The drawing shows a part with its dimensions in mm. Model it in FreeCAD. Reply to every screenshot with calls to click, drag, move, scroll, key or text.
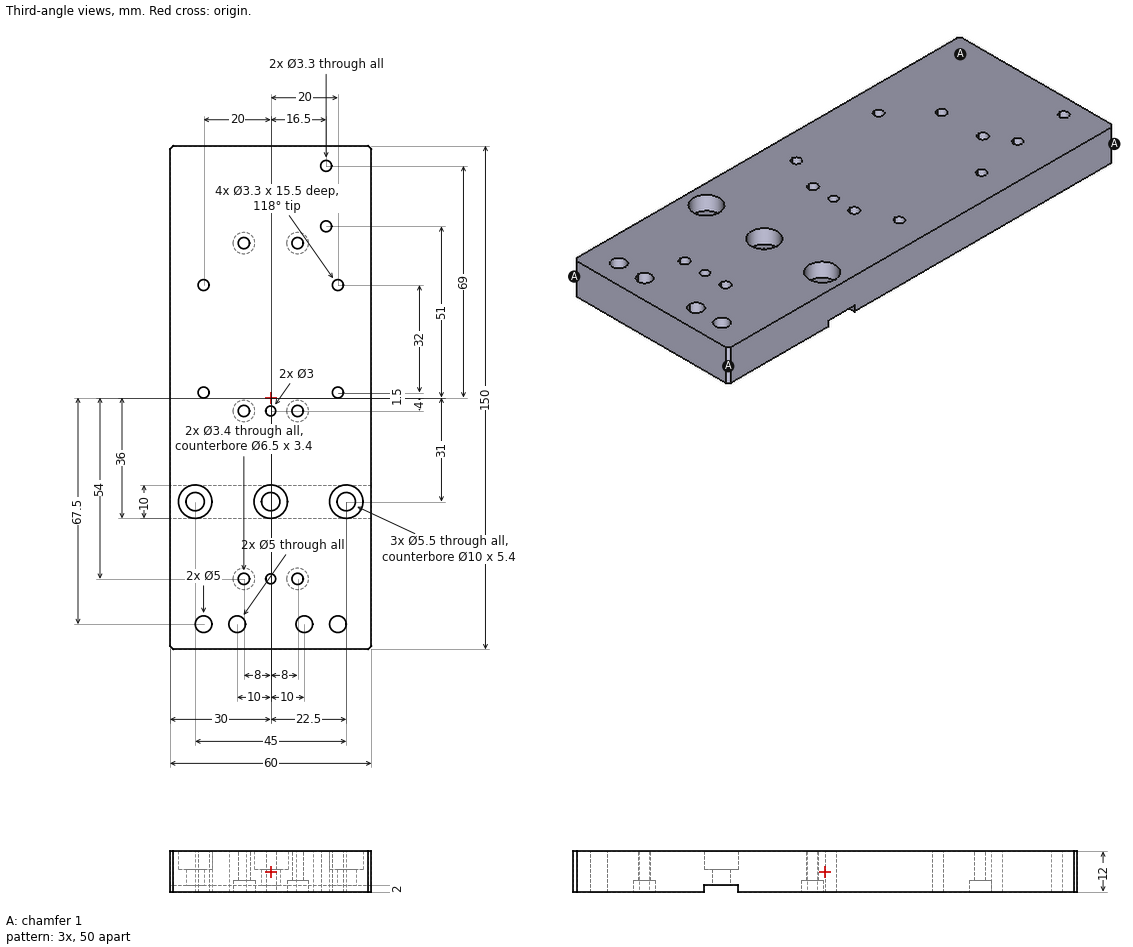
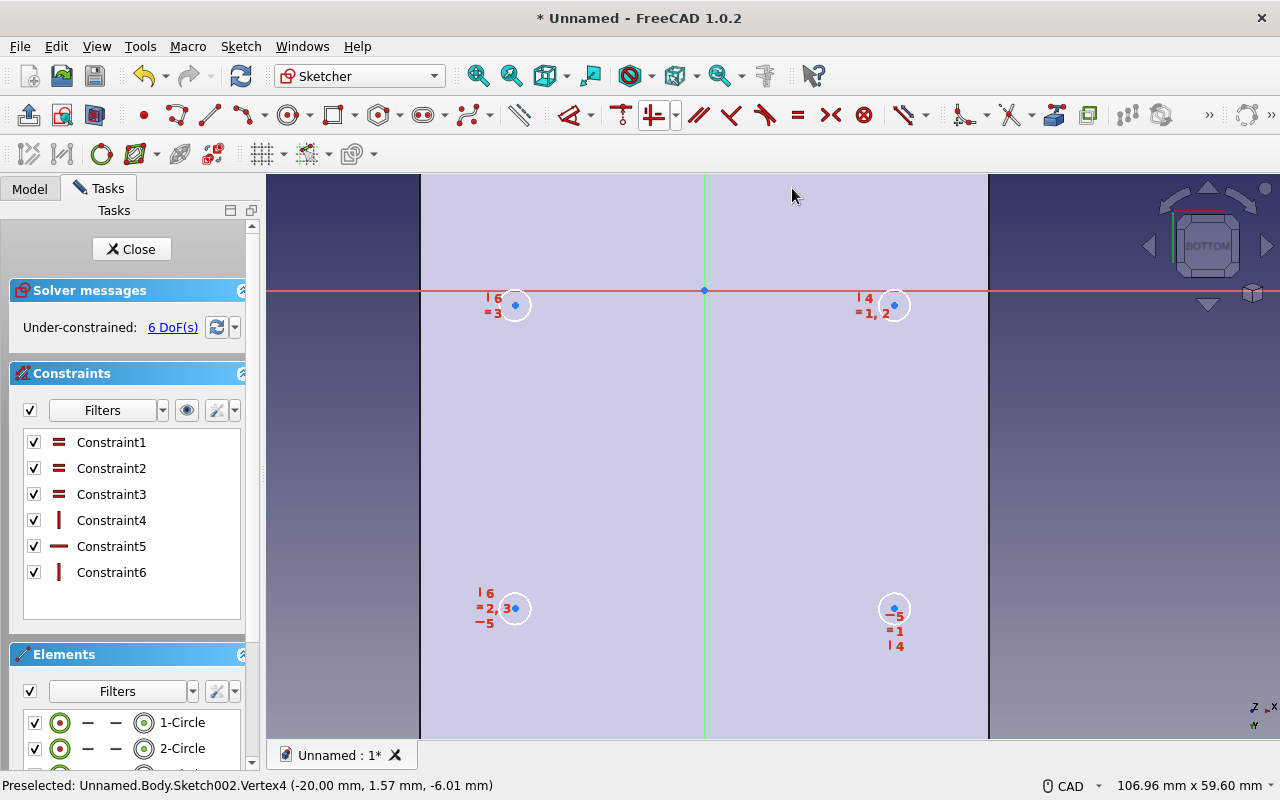
click(895, 305)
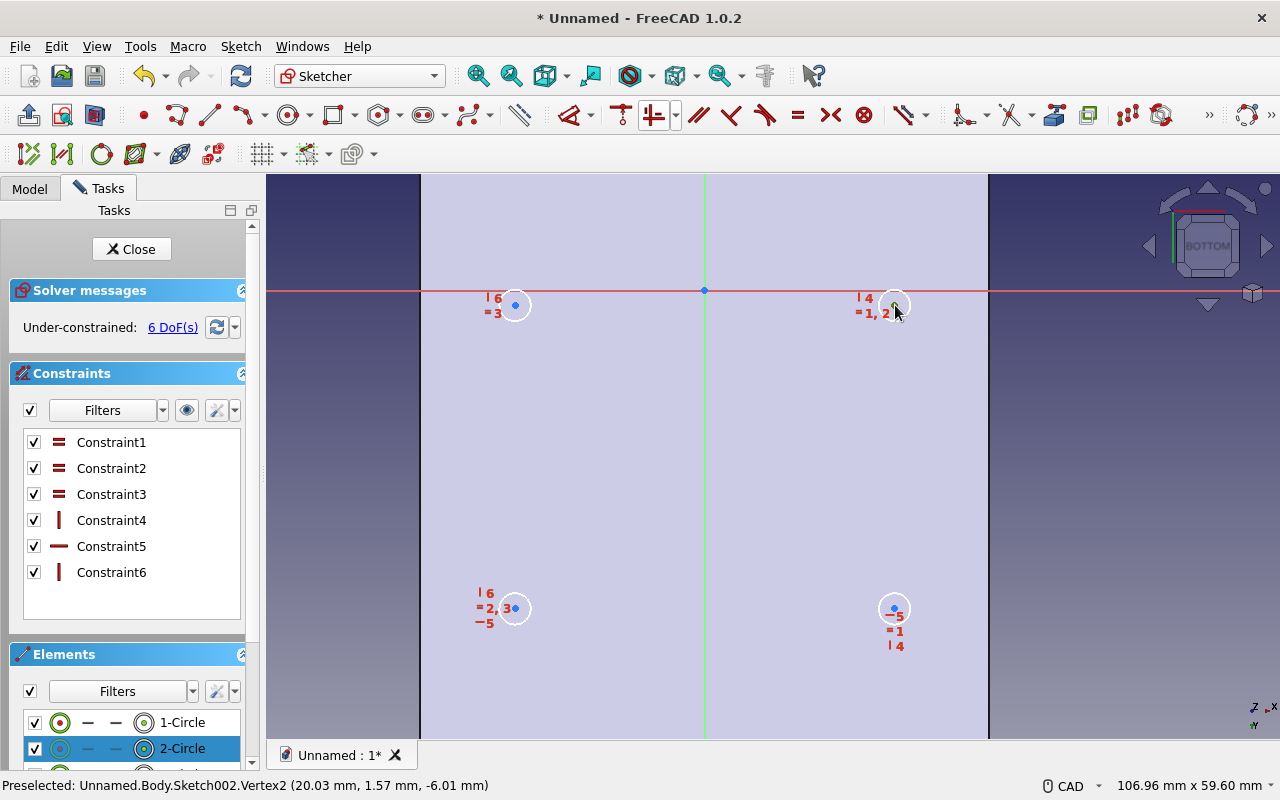
click(515, 305)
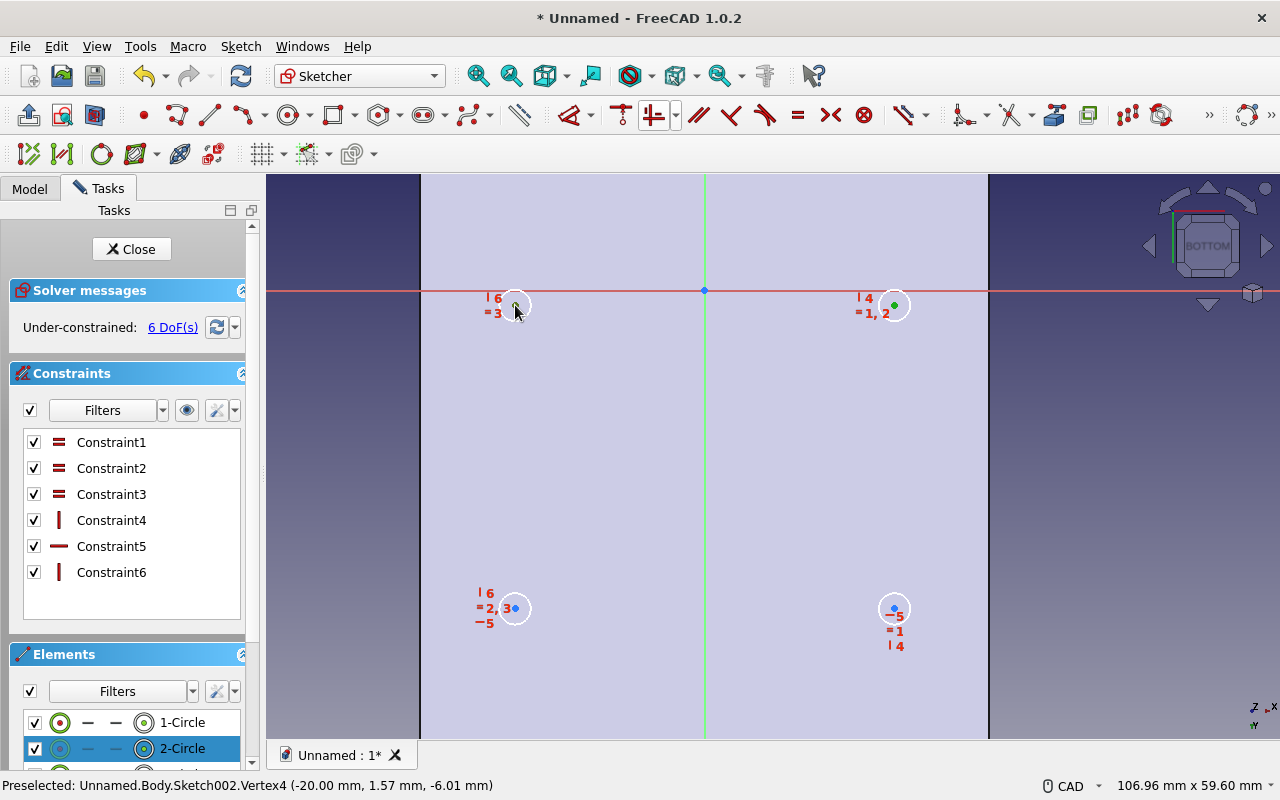
click(676, 116)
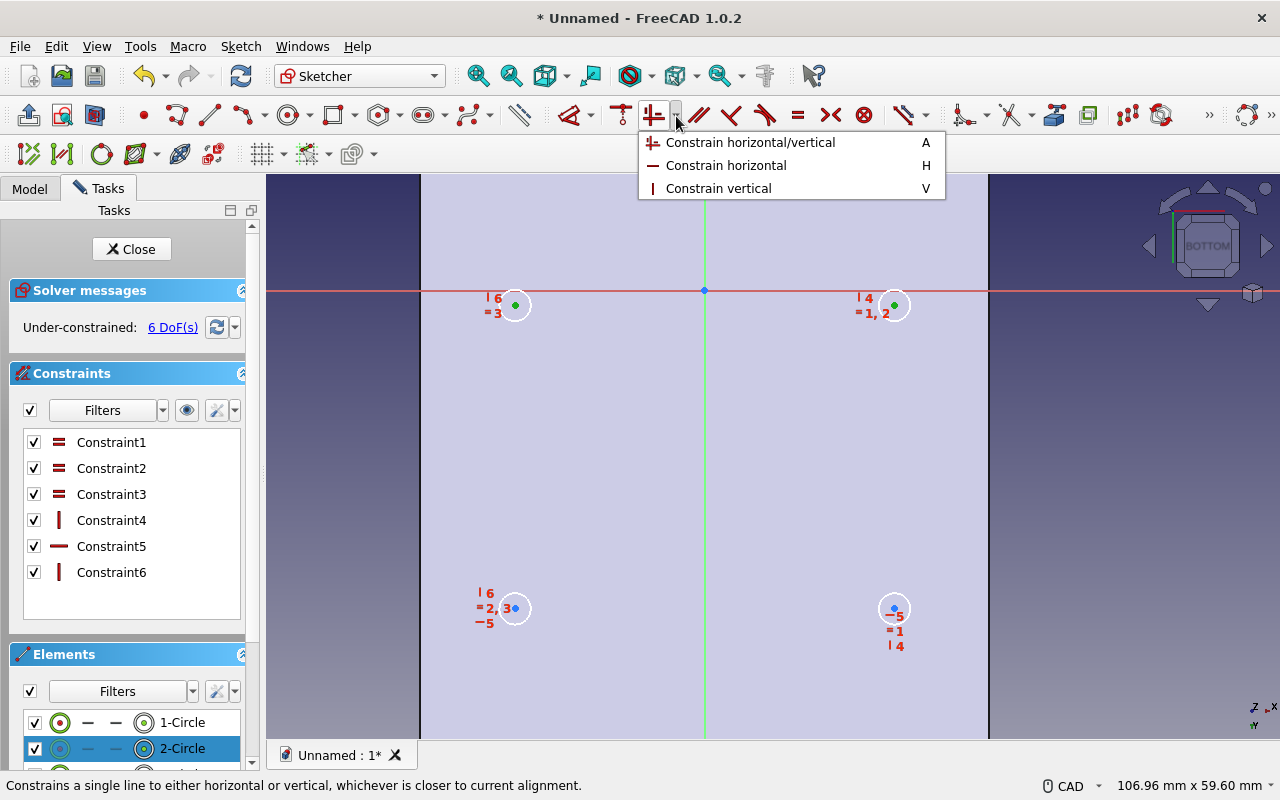
click(792, 166)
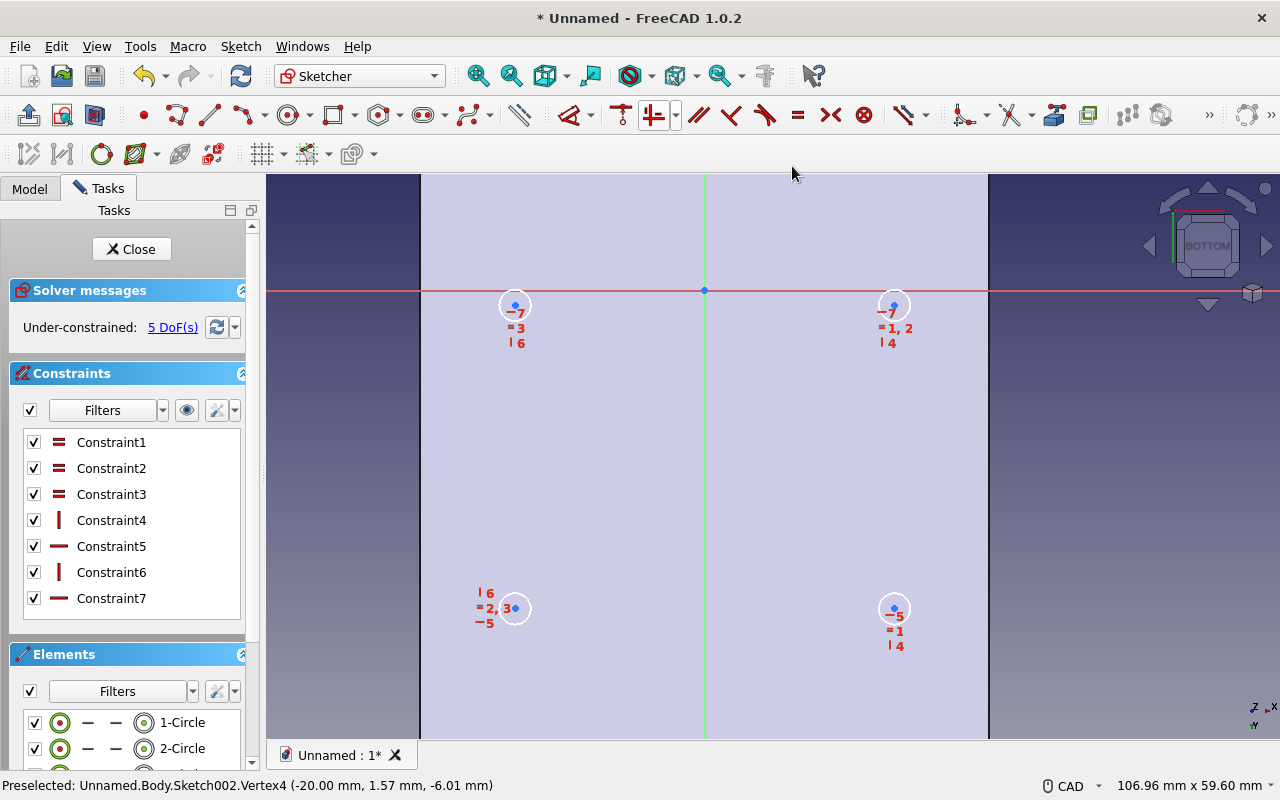
click(568, 116)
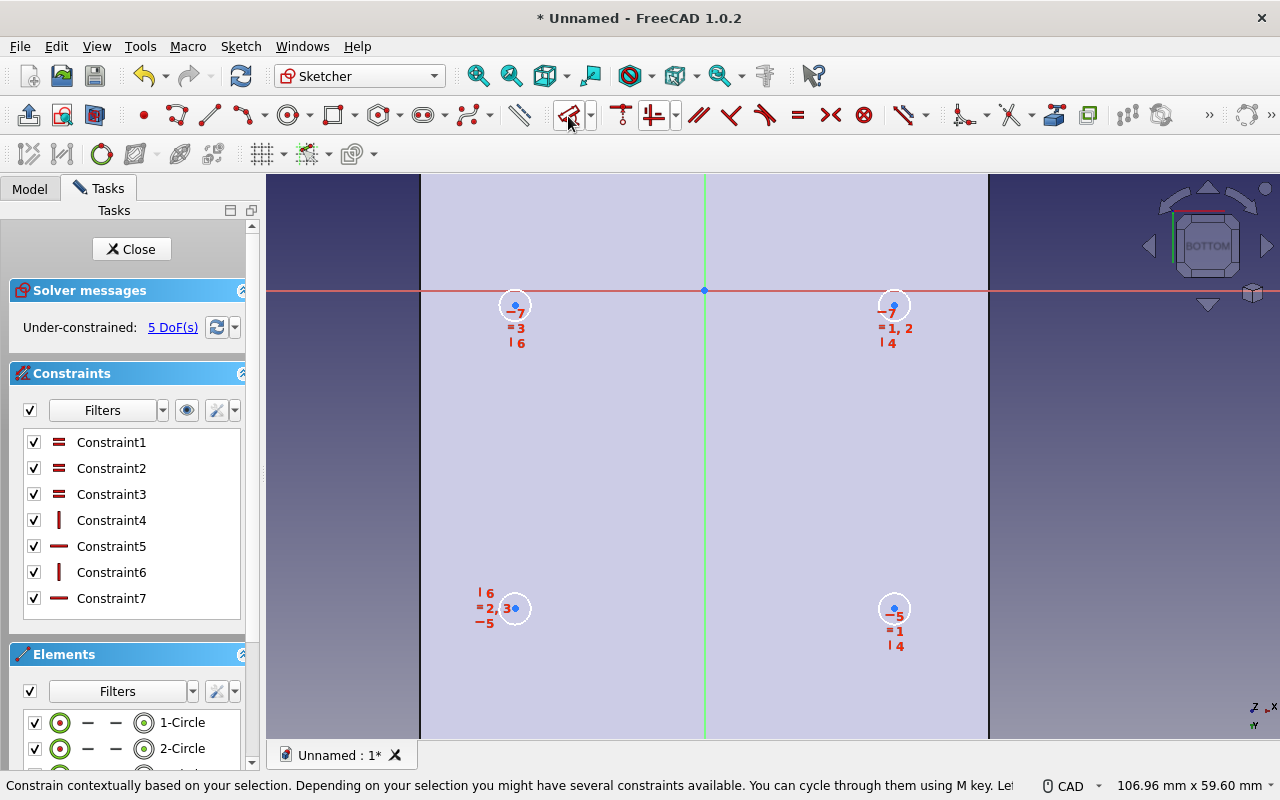
scroll(906, 598, up, 2)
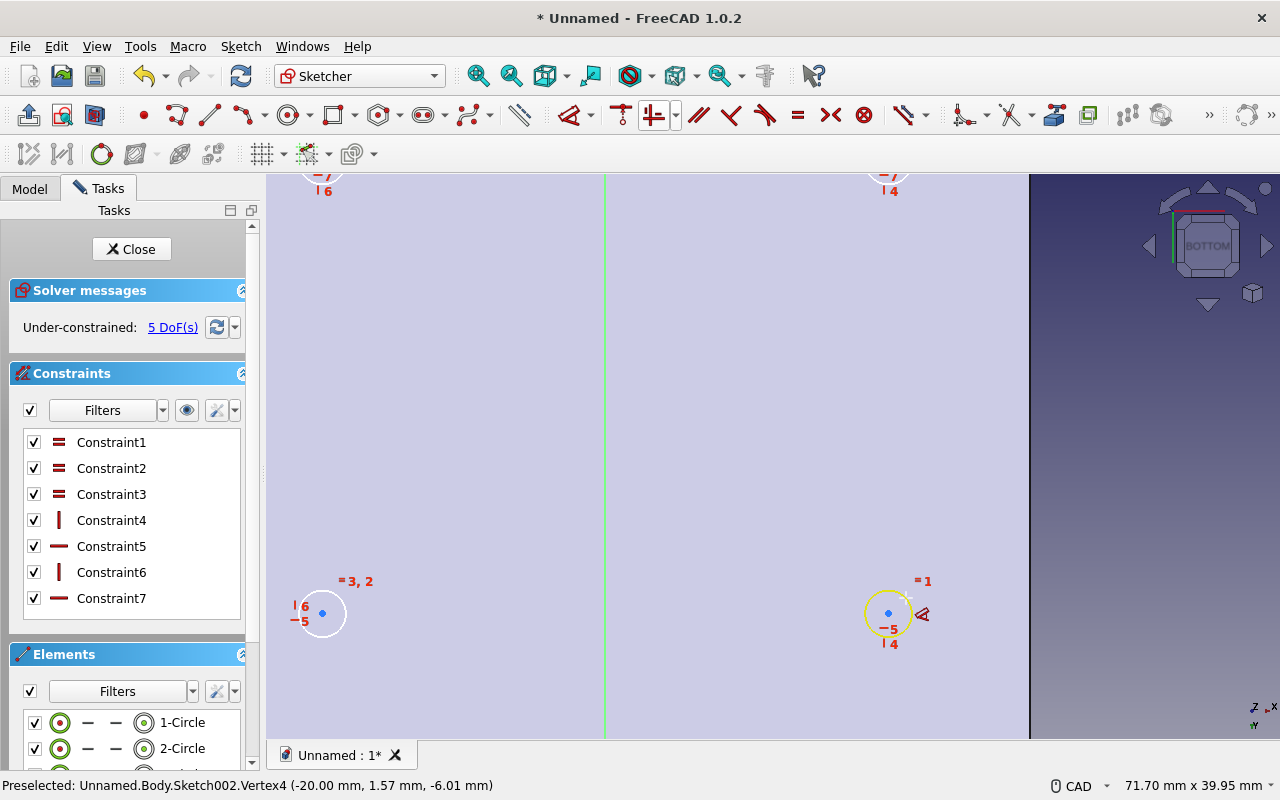
click(905, 597)
click(927, 574)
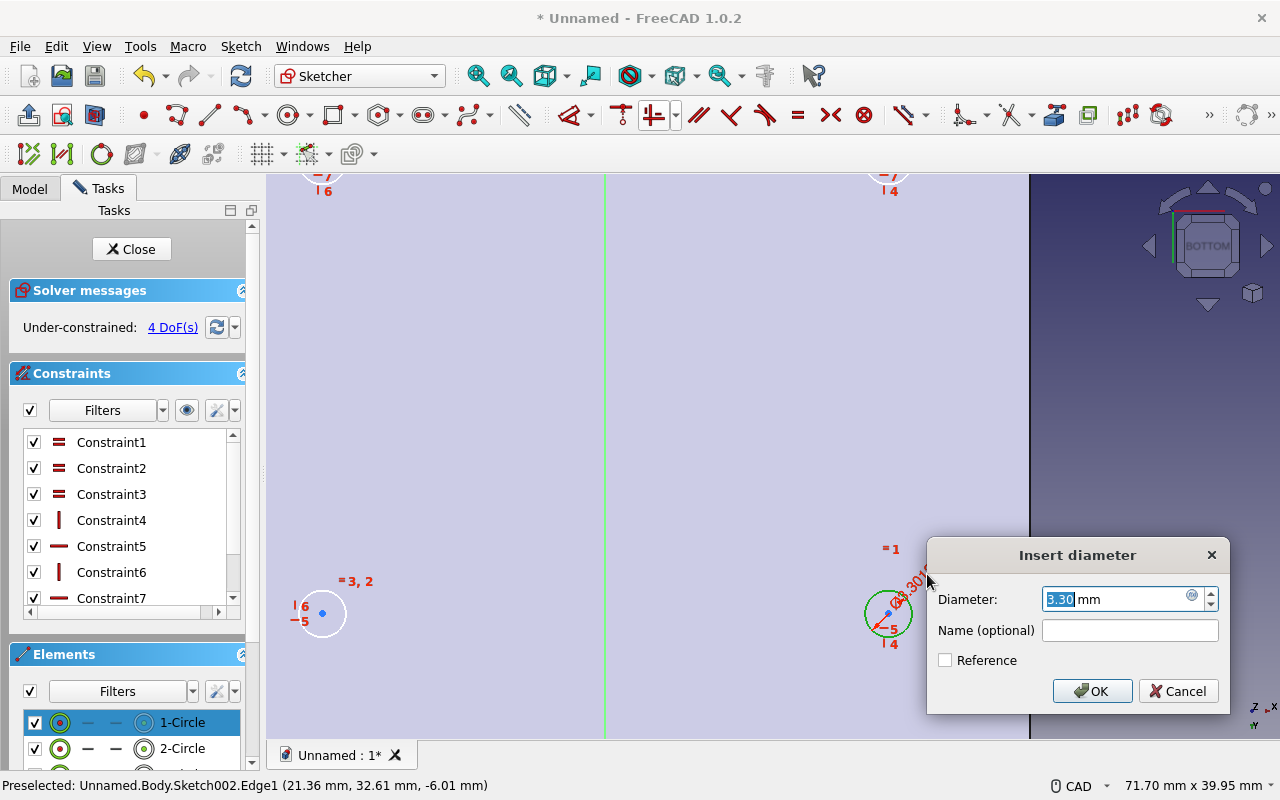
text(3.3)
key(Return)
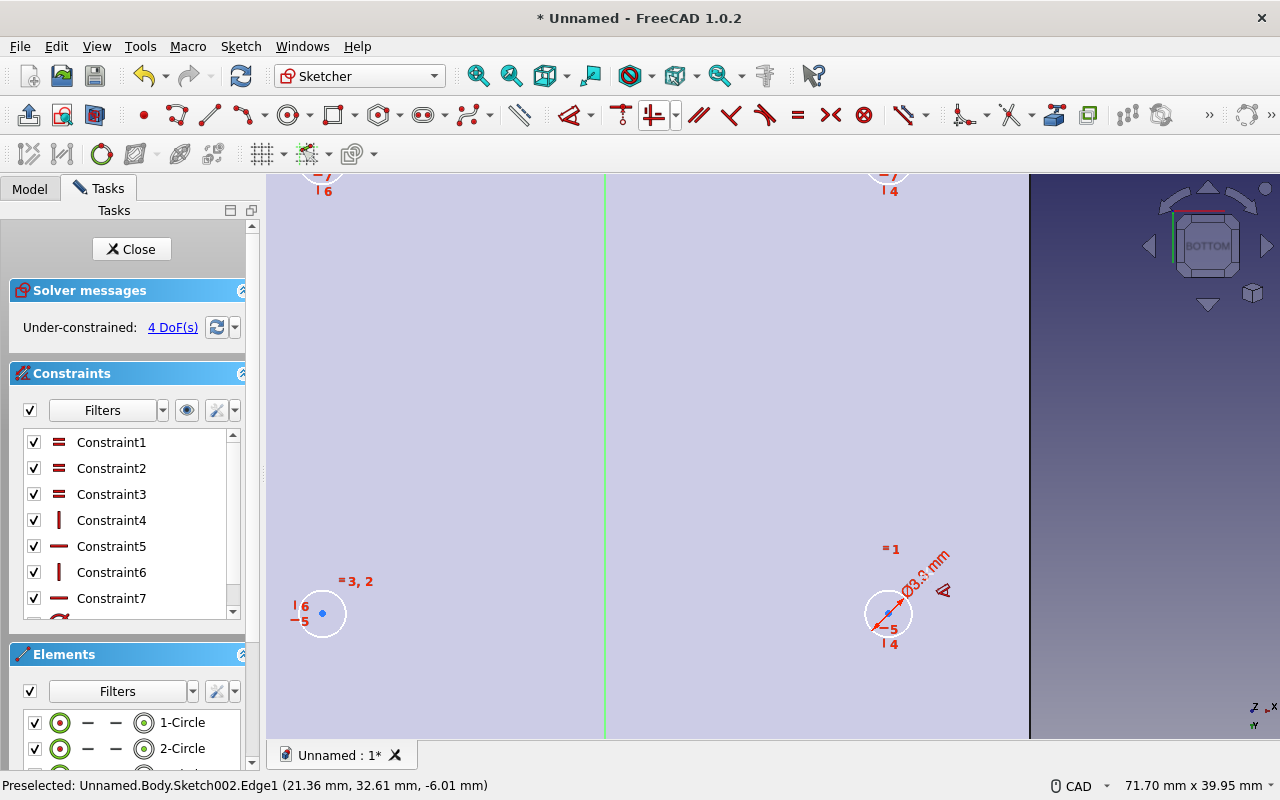
click(889, 614)
click(747, 648)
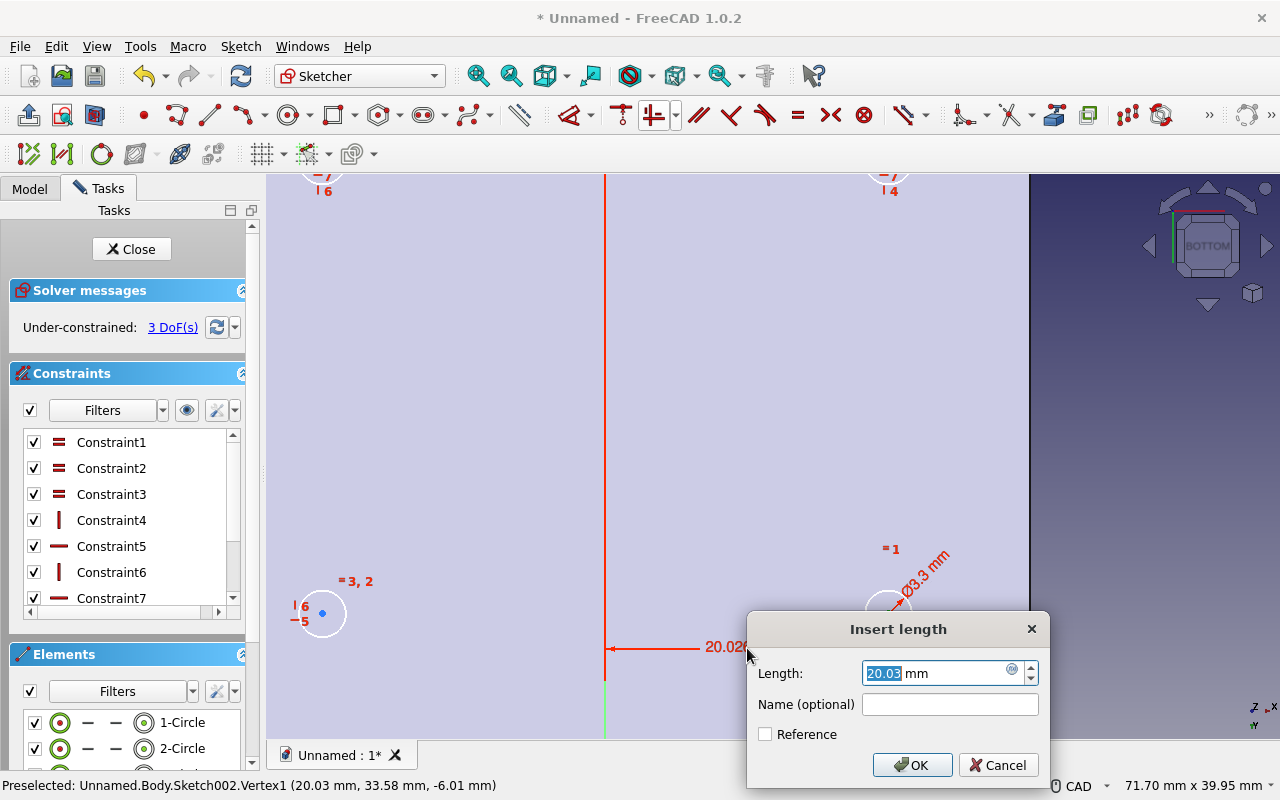
text(20)
key(Return)